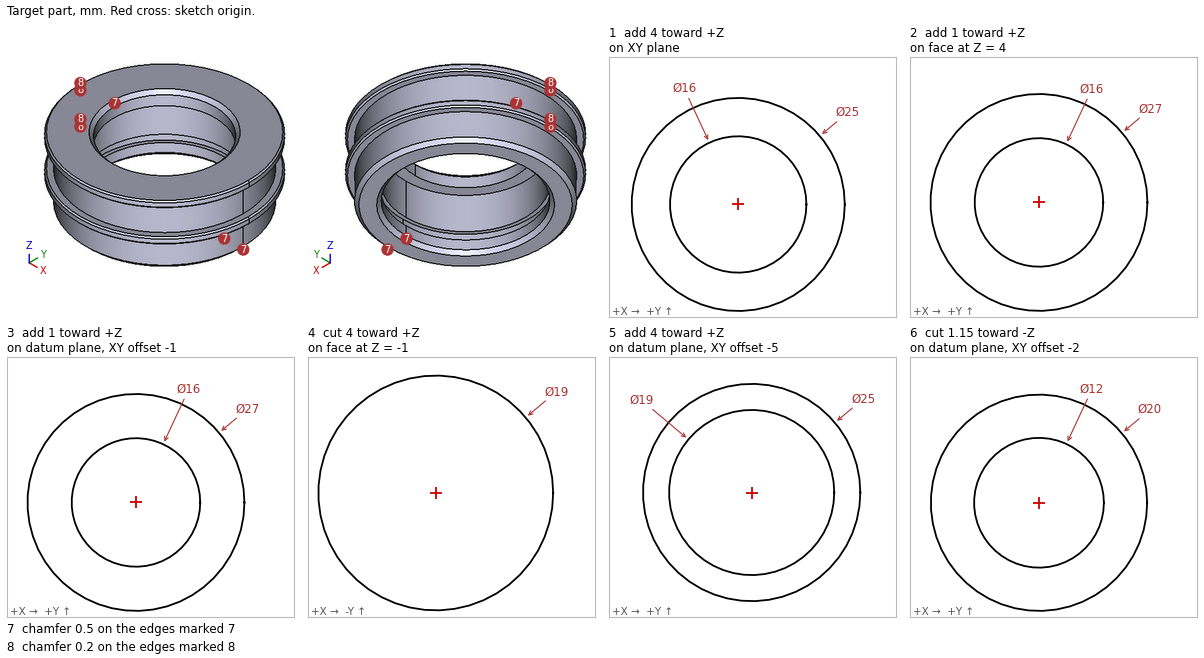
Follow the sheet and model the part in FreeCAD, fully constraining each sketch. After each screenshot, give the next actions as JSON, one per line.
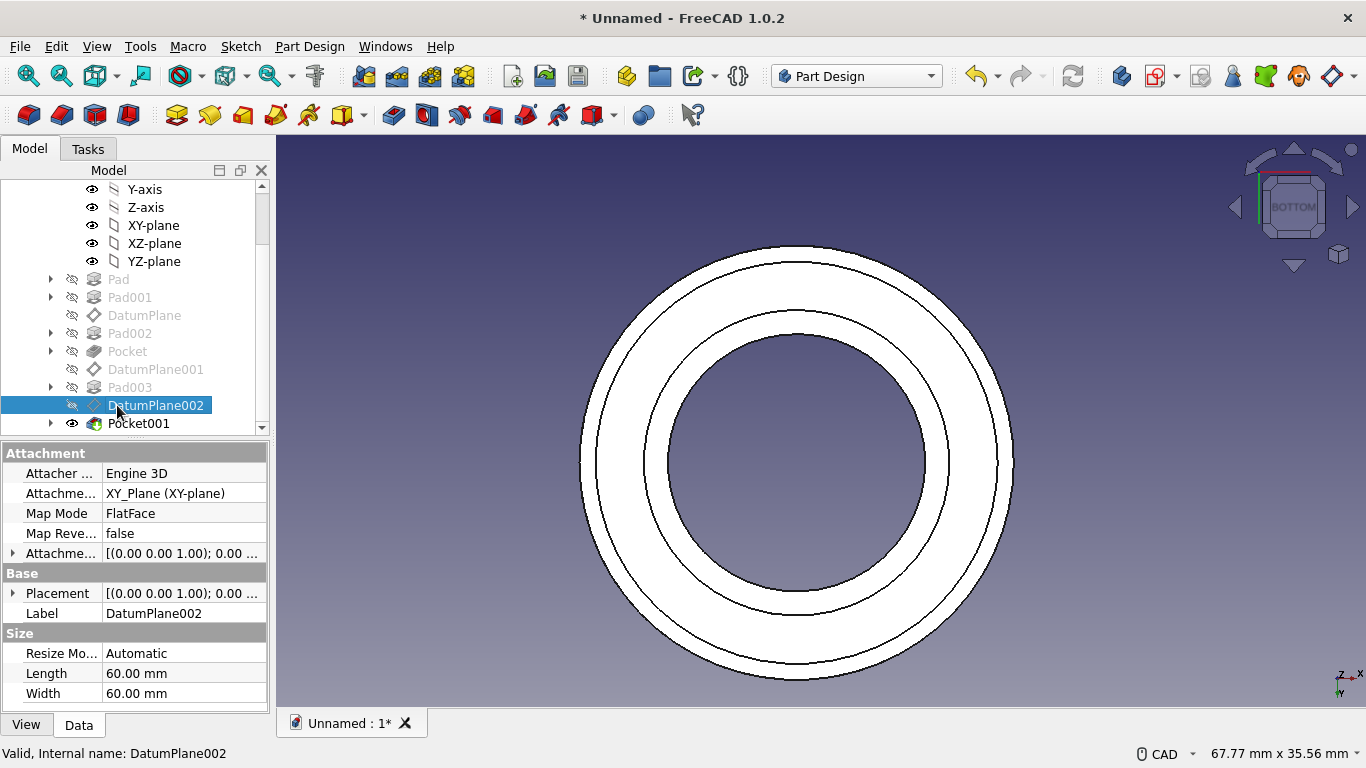
{"action": "left_click", "coordinate": [596, 462]}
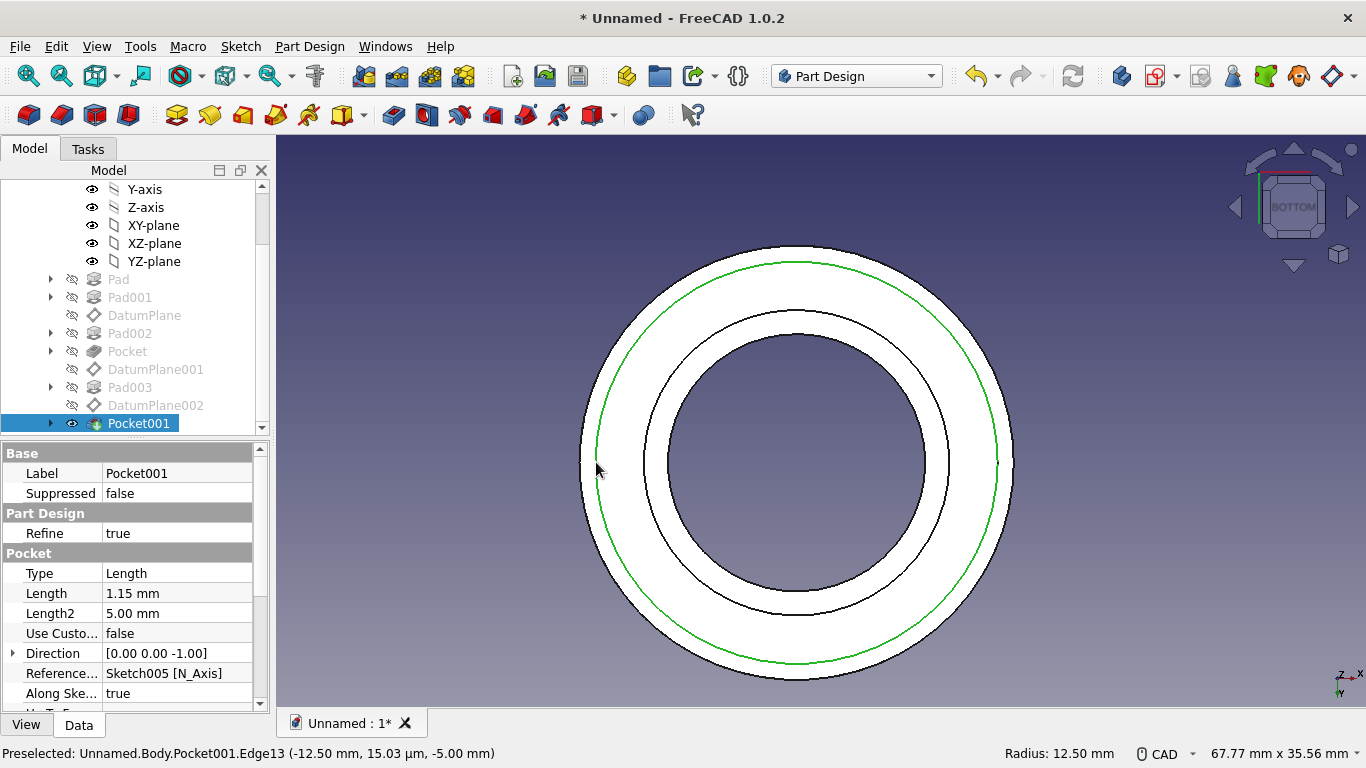
{"action": "left_click", "coordinate": [644, 462], "text": "ctrl"}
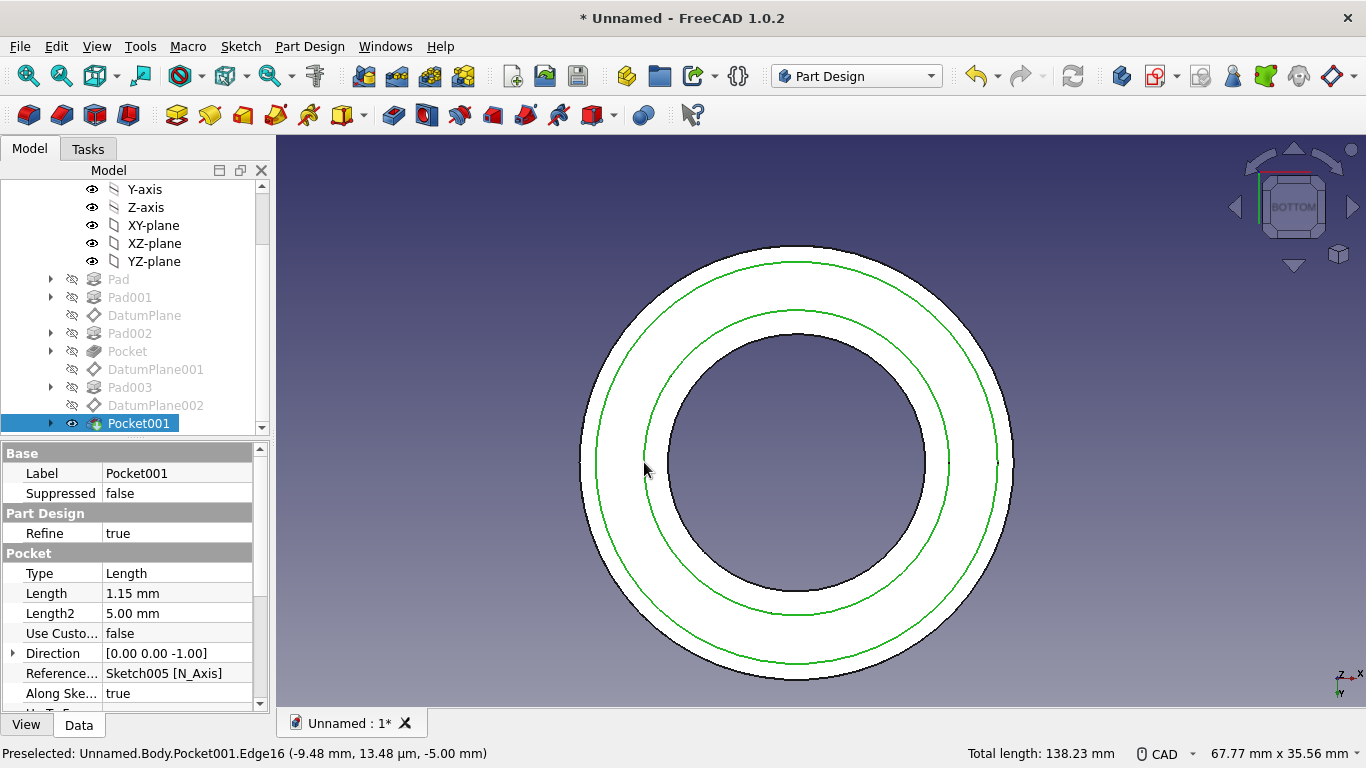
{"action": "key", "text": "0"}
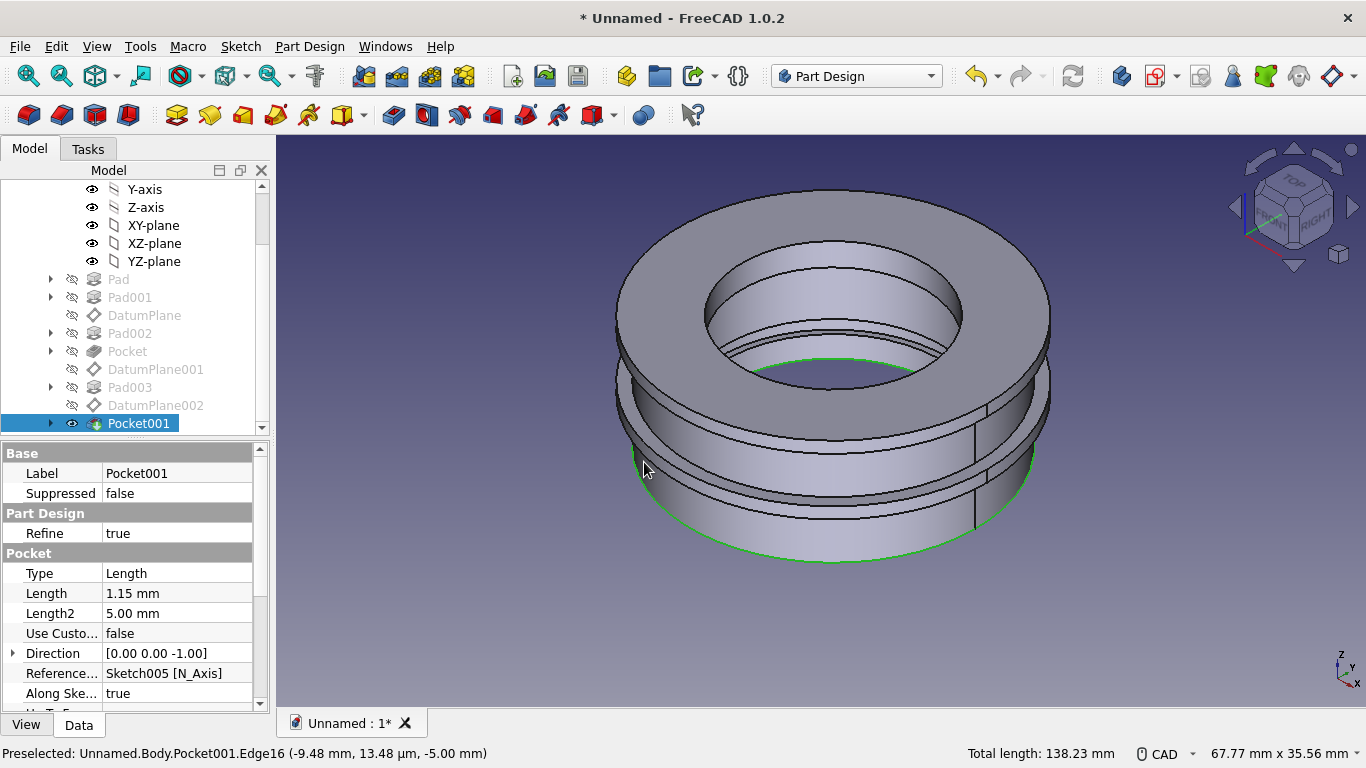
{"action": "left_click", "coordinate": [742, 262], "text": "ctrl"}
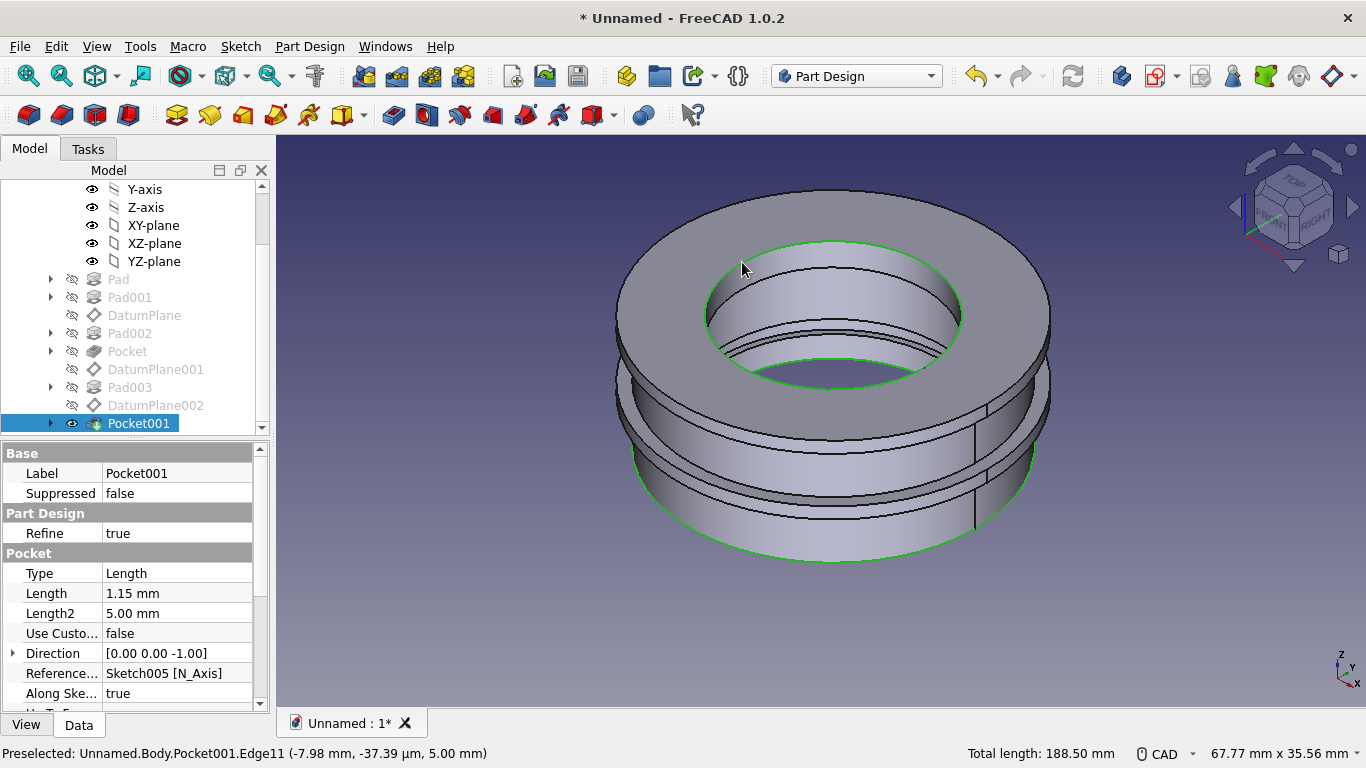
{"action": "left_click", "coordinate": [62, 116]}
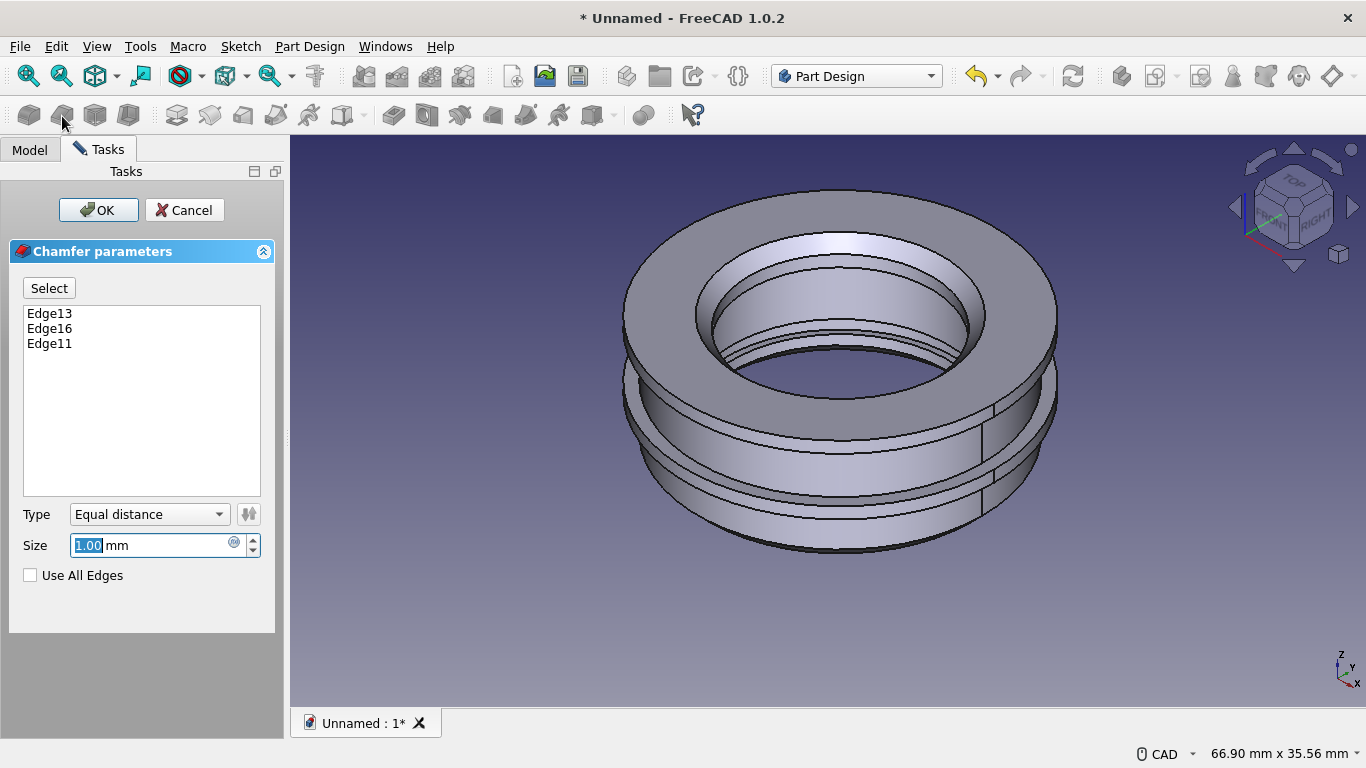
{"action": "type", "text": "0.5"}
{"action": "key", "text": "Tab"}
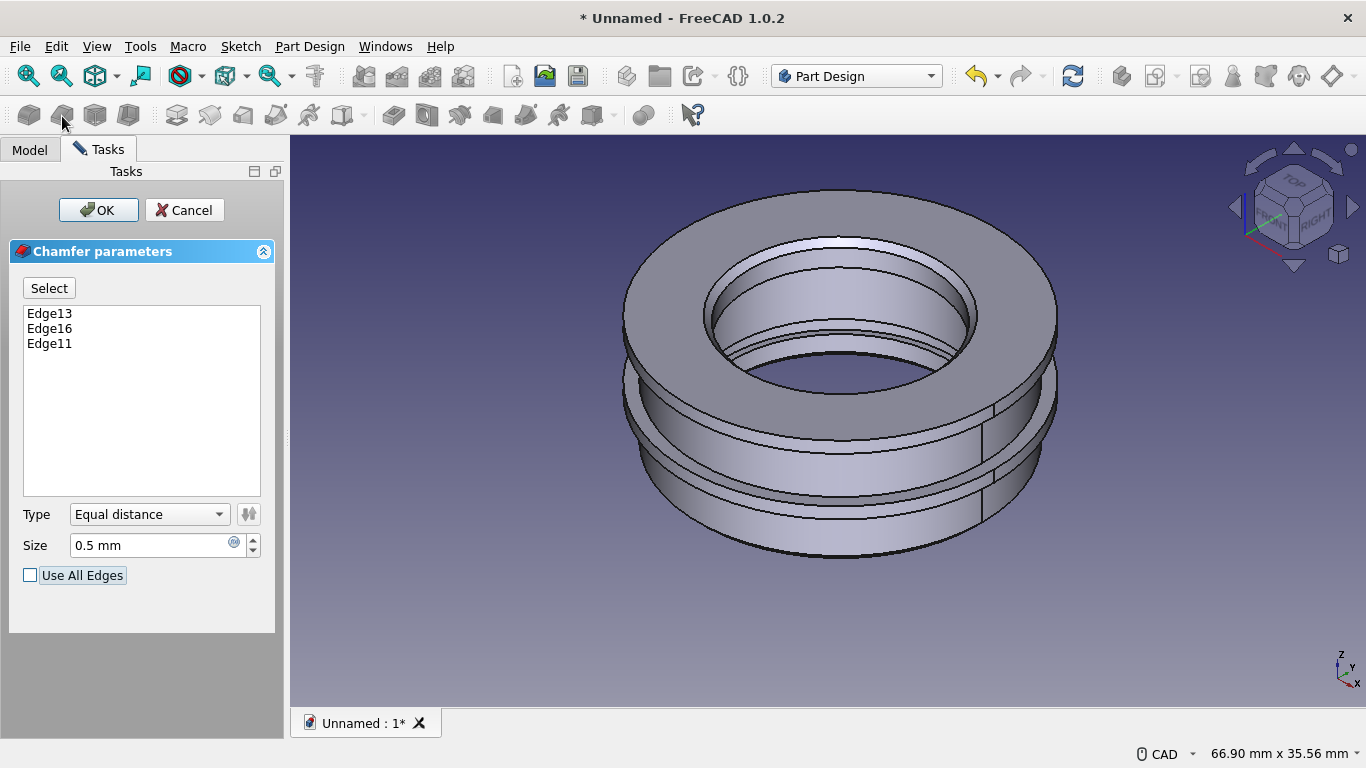
{"action": "left_click", "coordinate": [99, 210]}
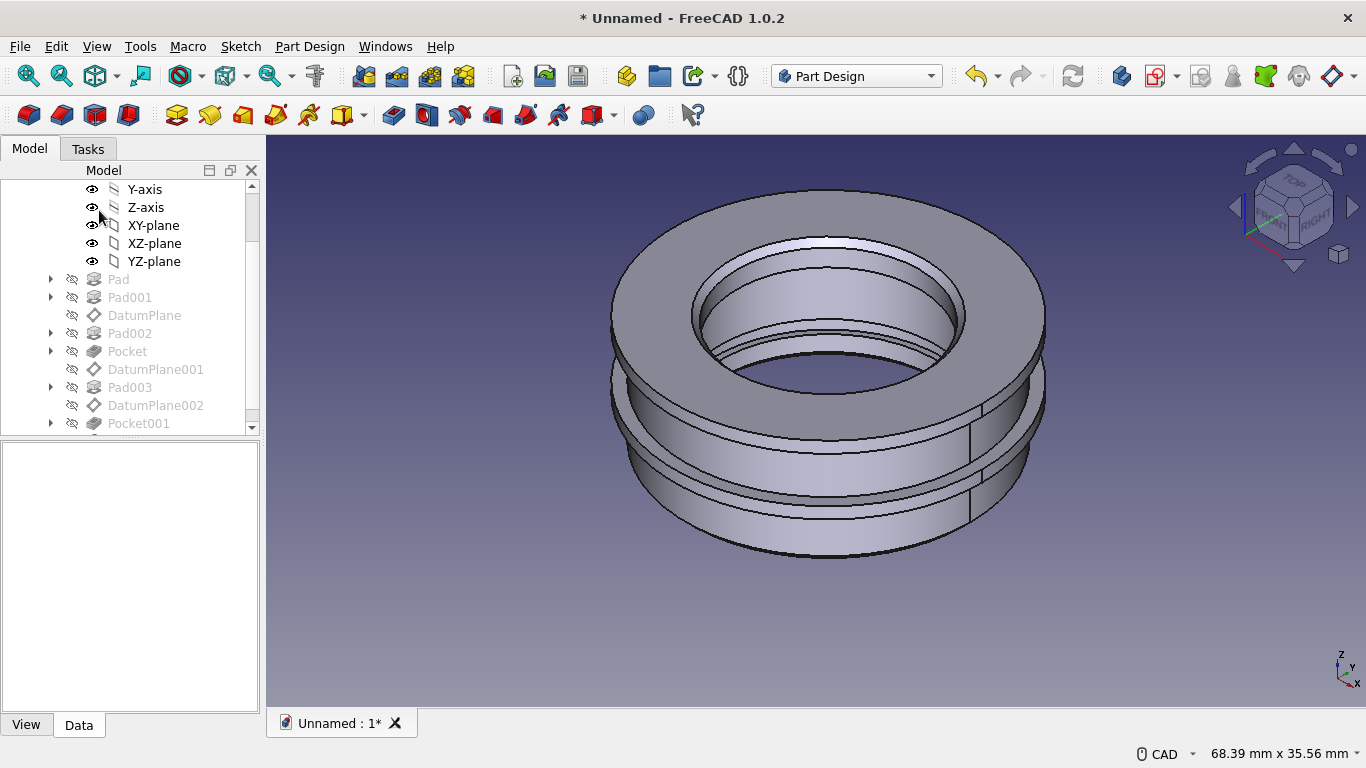
{"action": "left_click", "coordinate": [635, 437]}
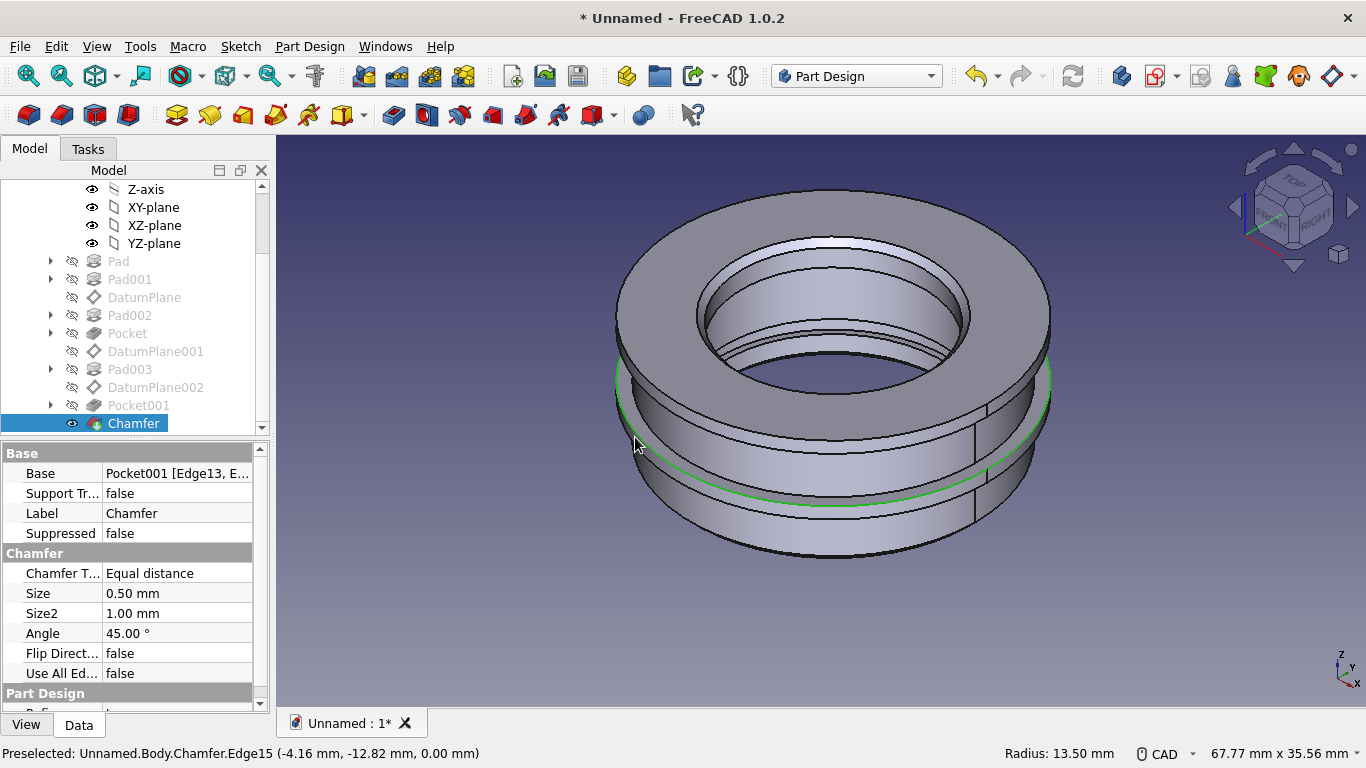
{"action": "left_click", "coordinate": [640, 371], "text": "ctrl"}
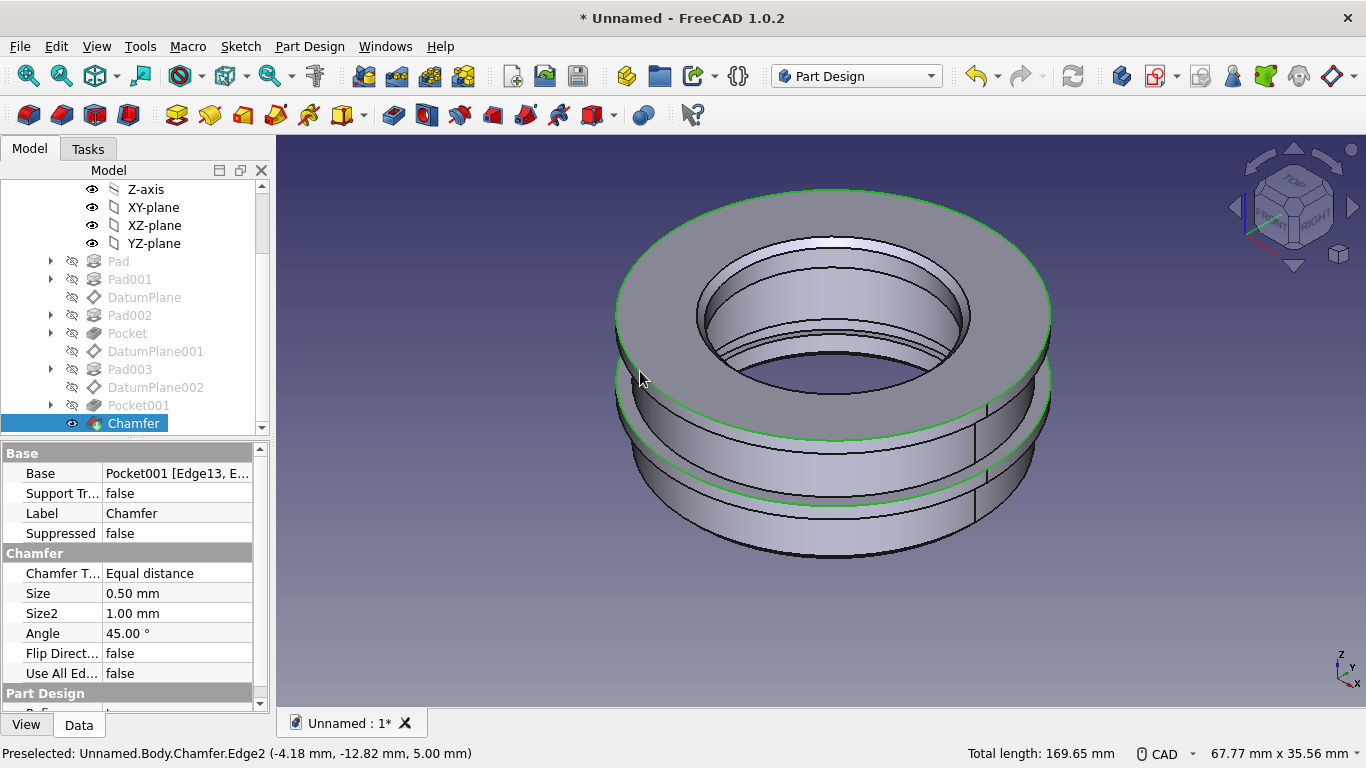
{"action": "key", "text": "2"}